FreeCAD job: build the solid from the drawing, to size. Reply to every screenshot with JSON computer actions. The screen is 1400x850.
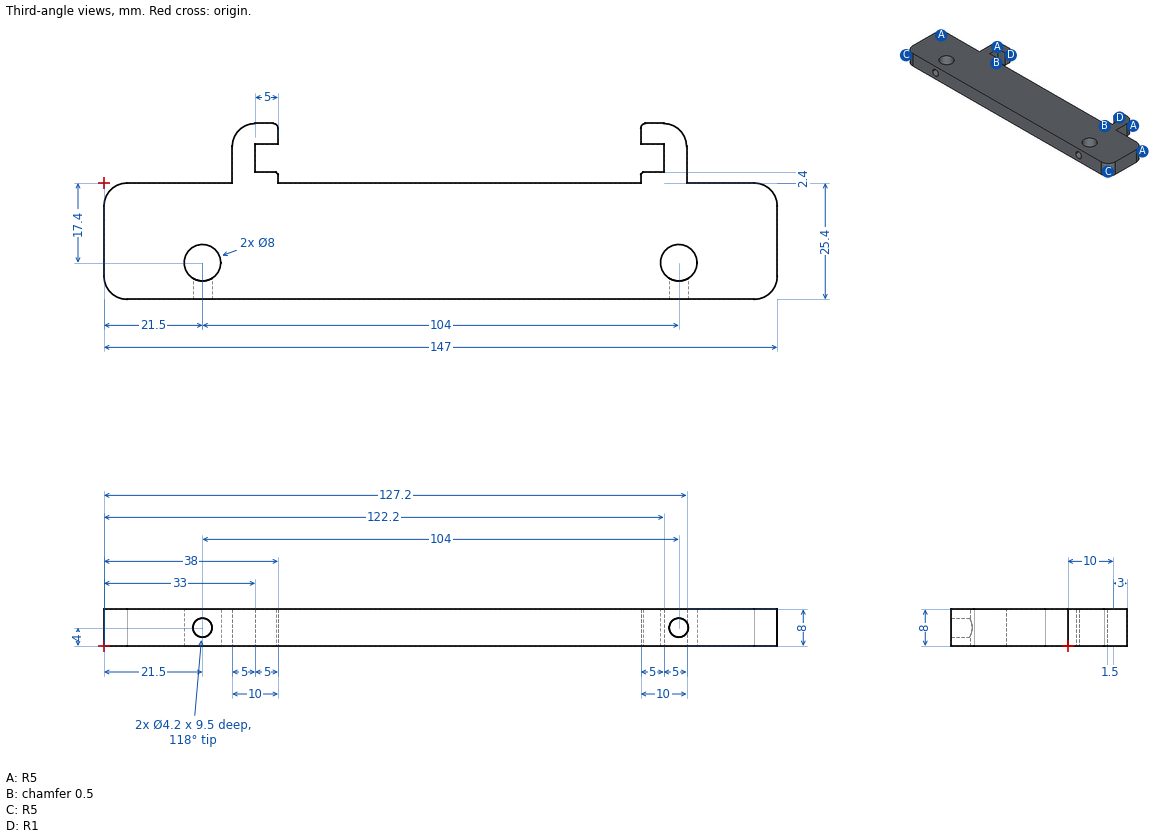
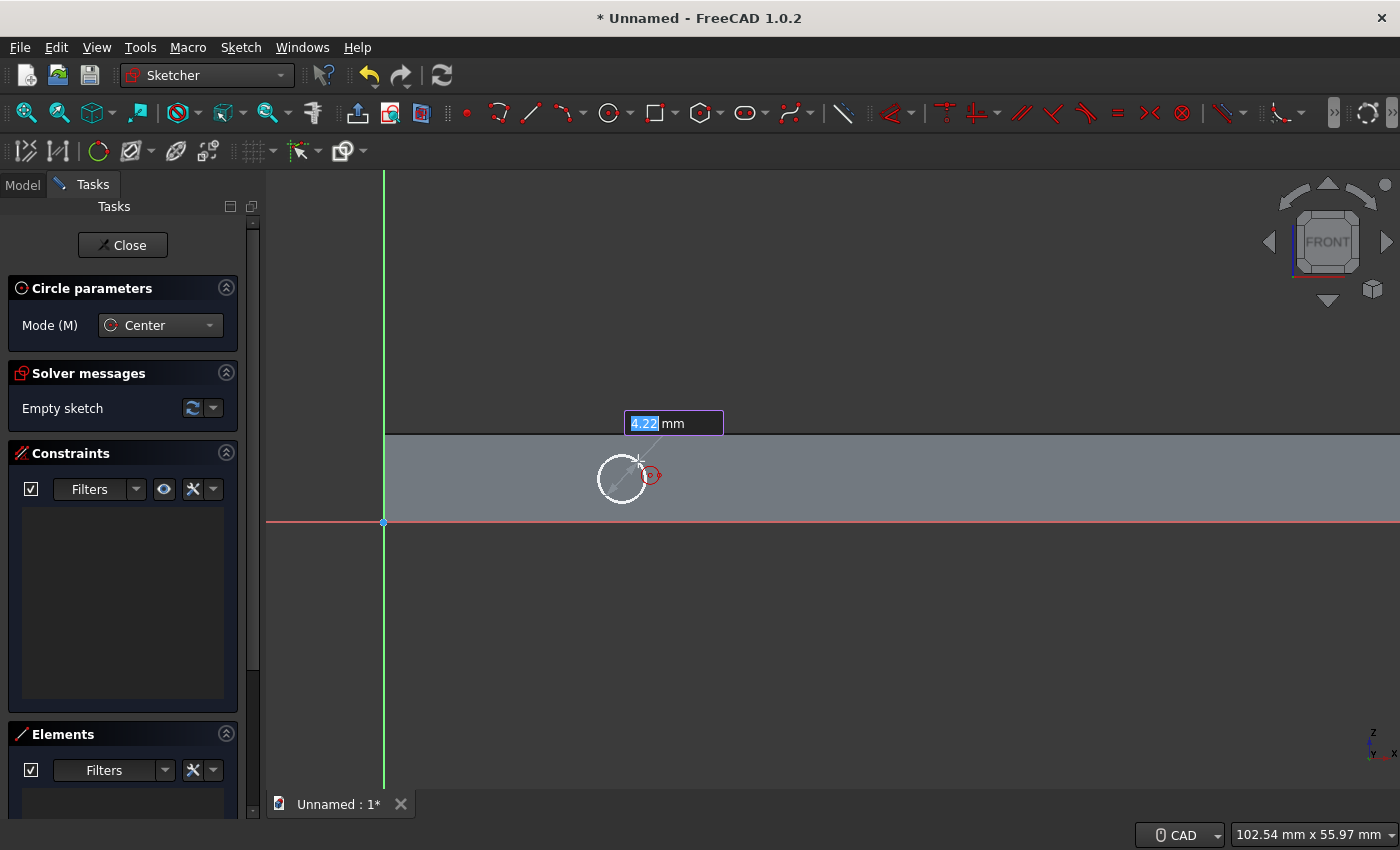
{"action": "type", "text": "4.2"}
{"action": "key", "text": "Return"}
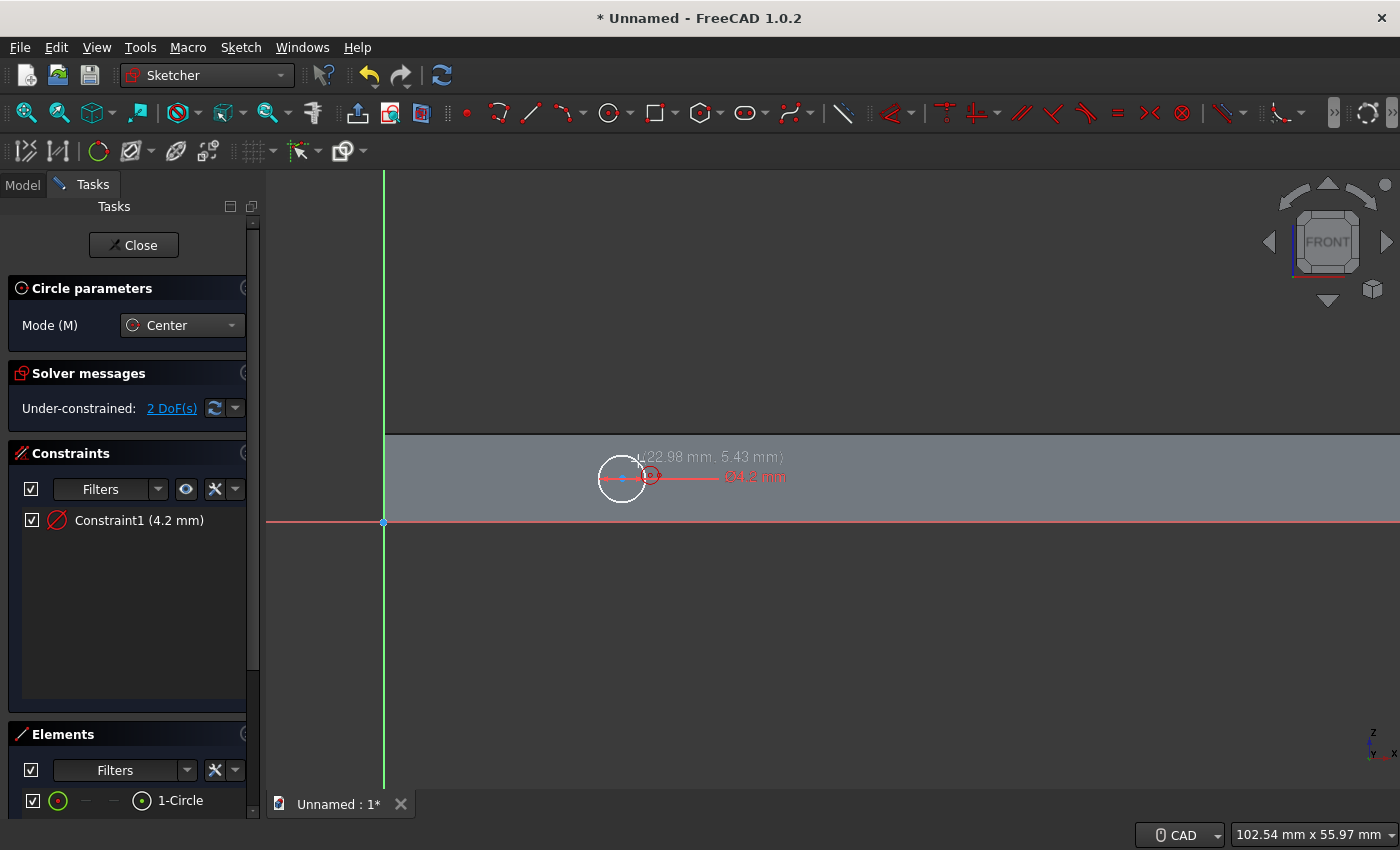
{"action": "scroll", "coordinate": [499, 472], "scroll_direction": "down", "scroll_amount": 4}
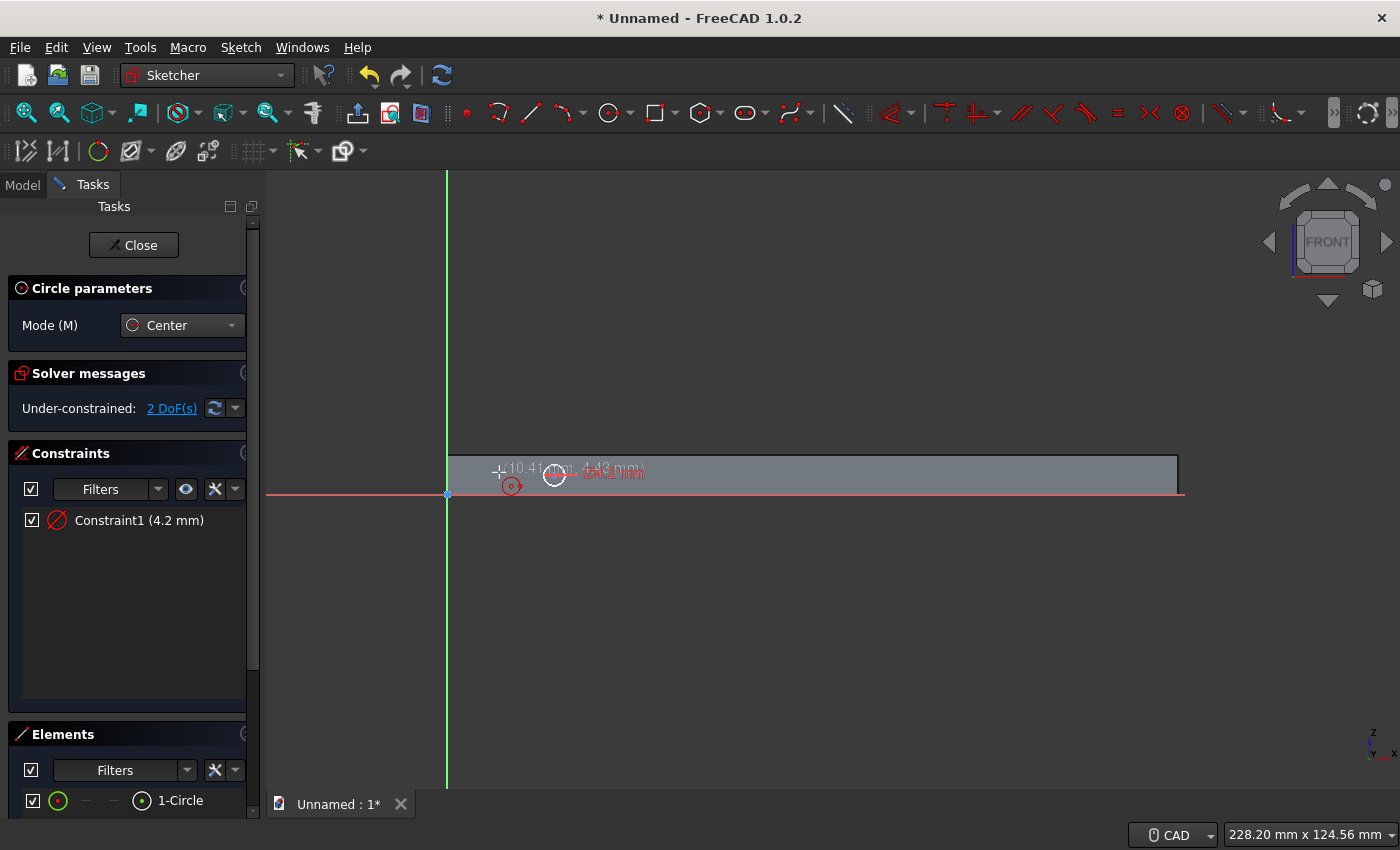
{"action": "scroll", "coordinate": [1071, 475], "scroll_direction": "up", "scroll_amount": 4}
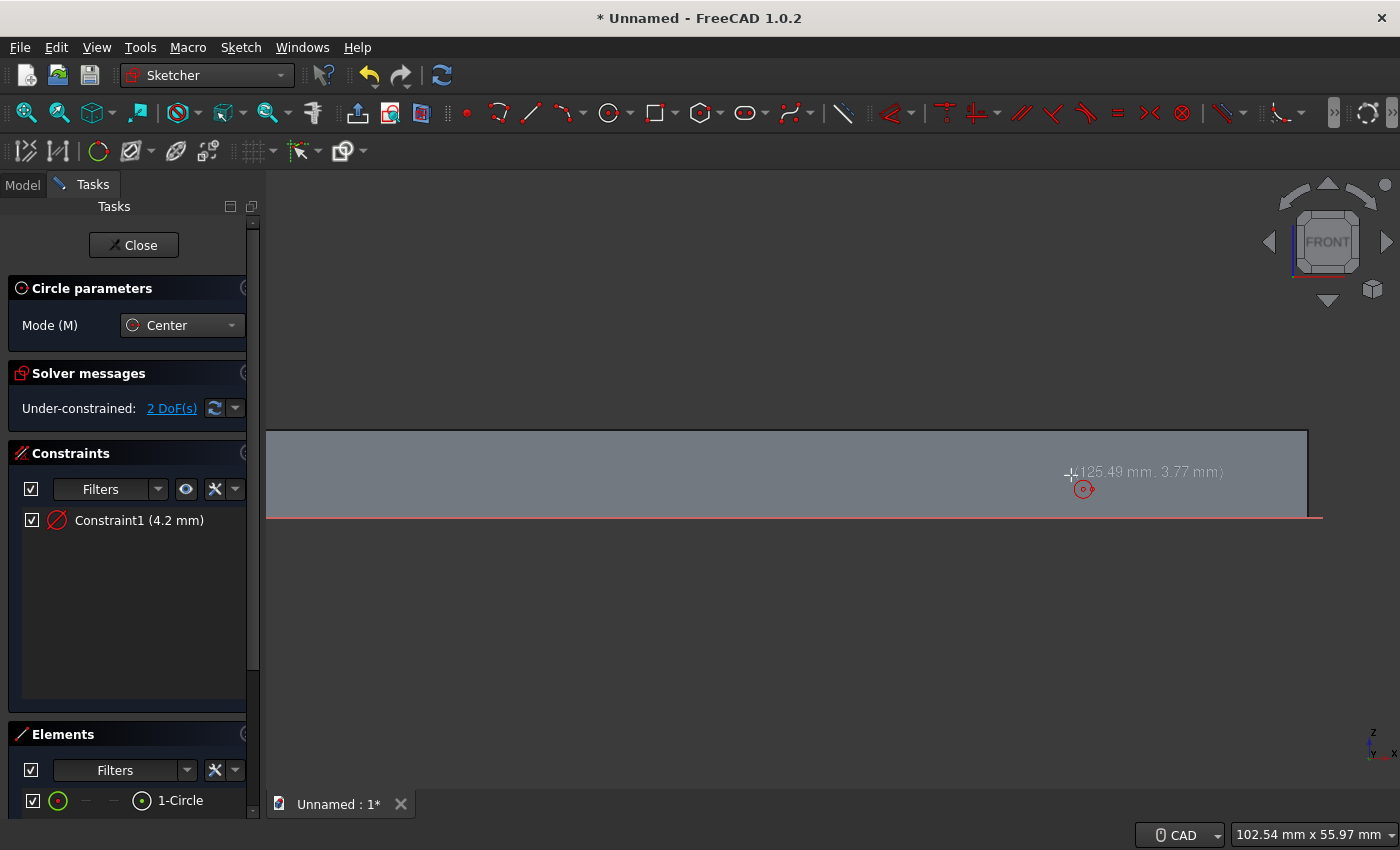
{"action": "left_click", "coordinate": [1070, 474]}
{"action": "mouse_move", "coordinate": [1087, 458]}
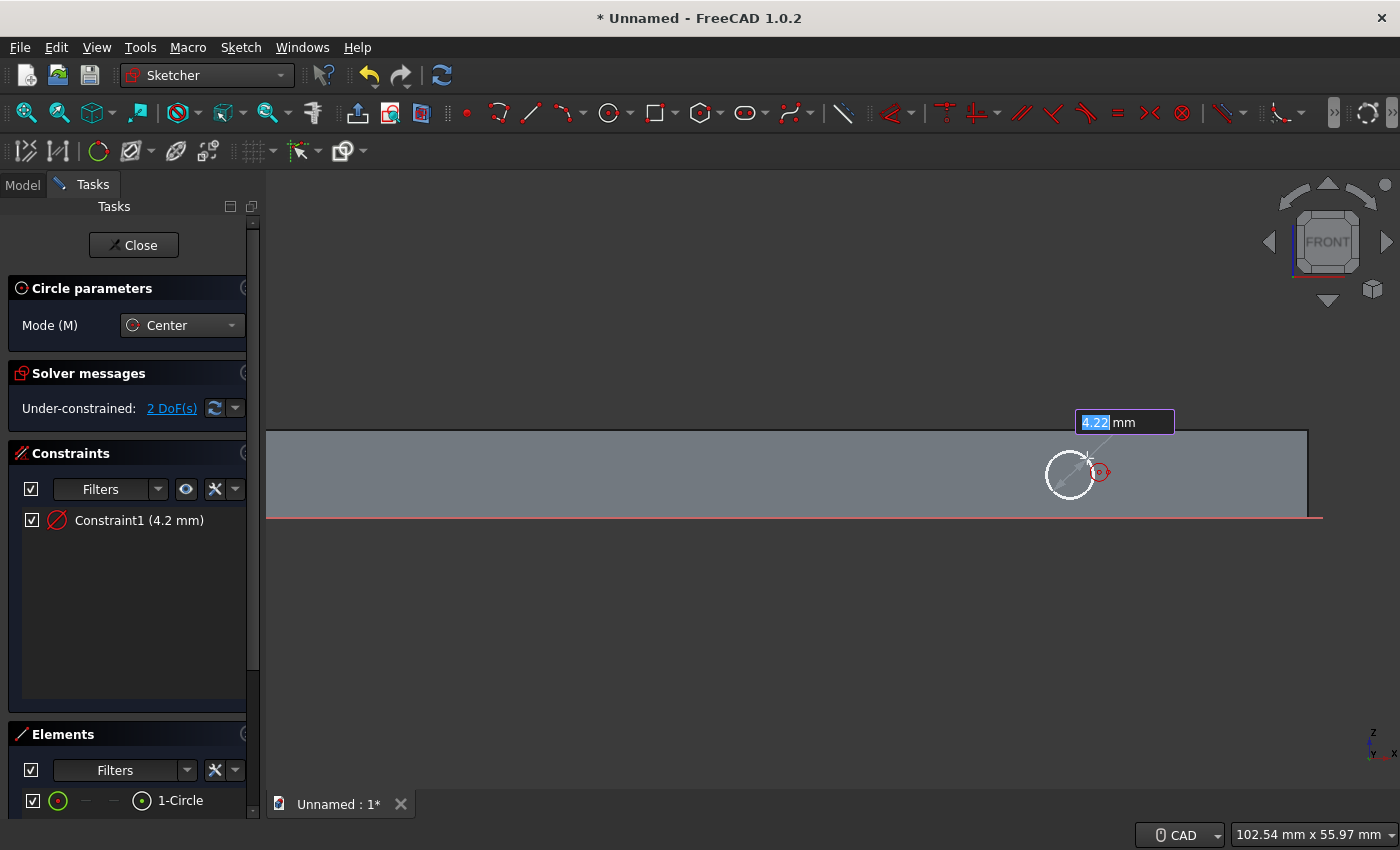
{"action": "type", "text": "4.2"}
{"action": "key", "text": "Return"}
{"action": "key", "text": "Escape"}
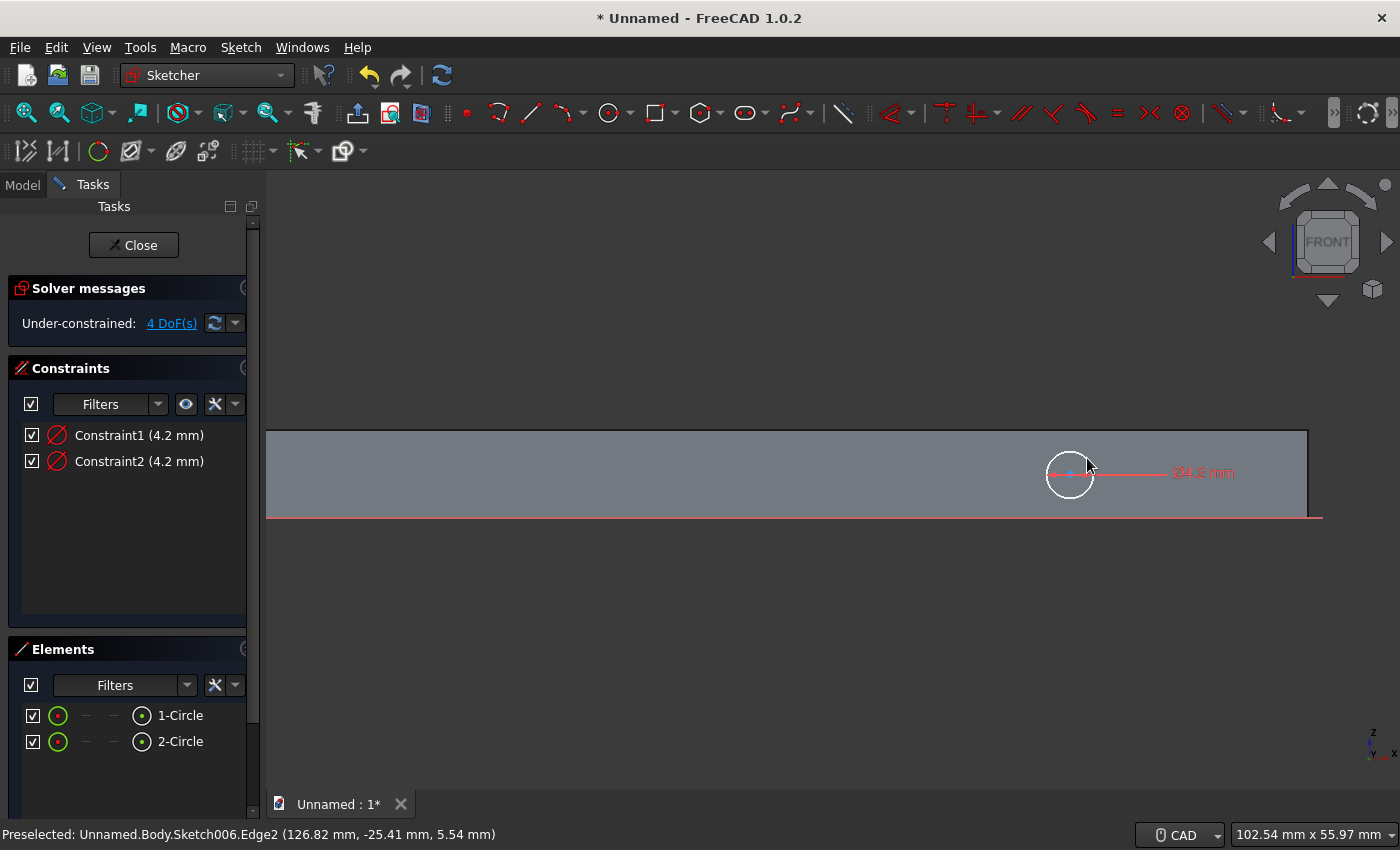
{"action": "left_click", "coordinate": [890, 114]}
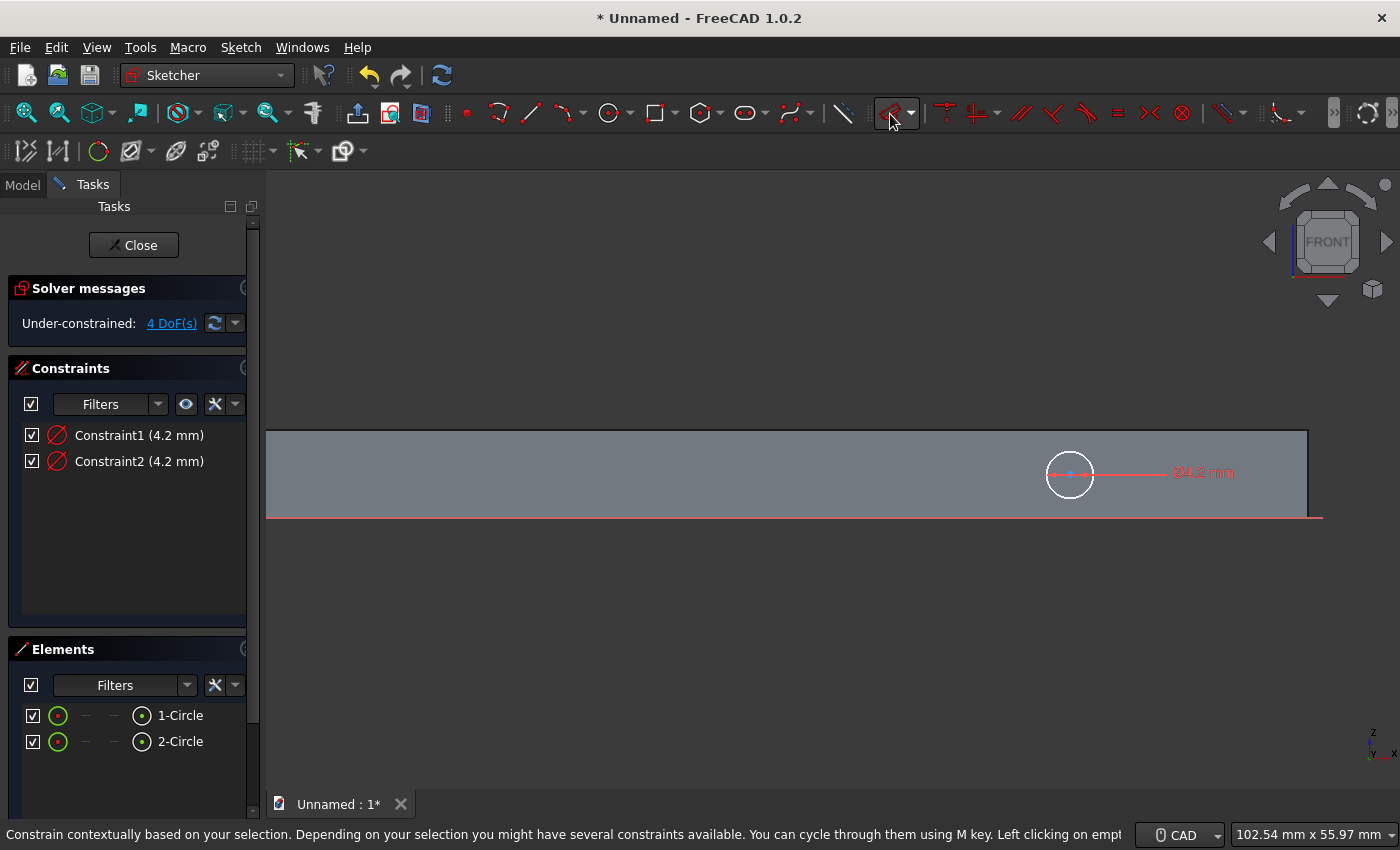
{"action": "scroll", "coordinate": [1072, 475], "scroll_direction": "down", "scroll_amount": 4}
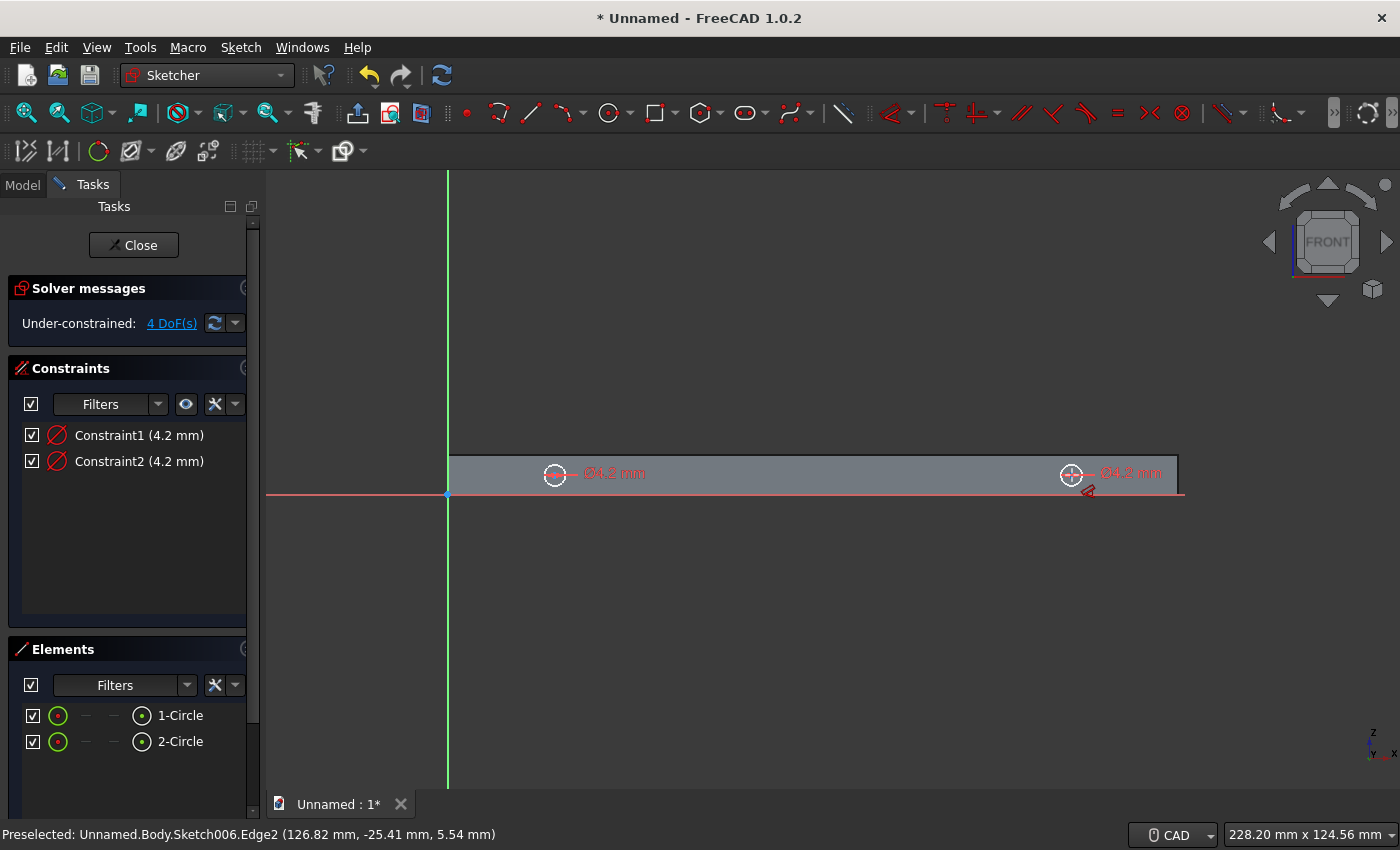
{"action": "scroll", "coordinate": [555, 475], "scroll_direction": "up", "scroll_amount": 4}